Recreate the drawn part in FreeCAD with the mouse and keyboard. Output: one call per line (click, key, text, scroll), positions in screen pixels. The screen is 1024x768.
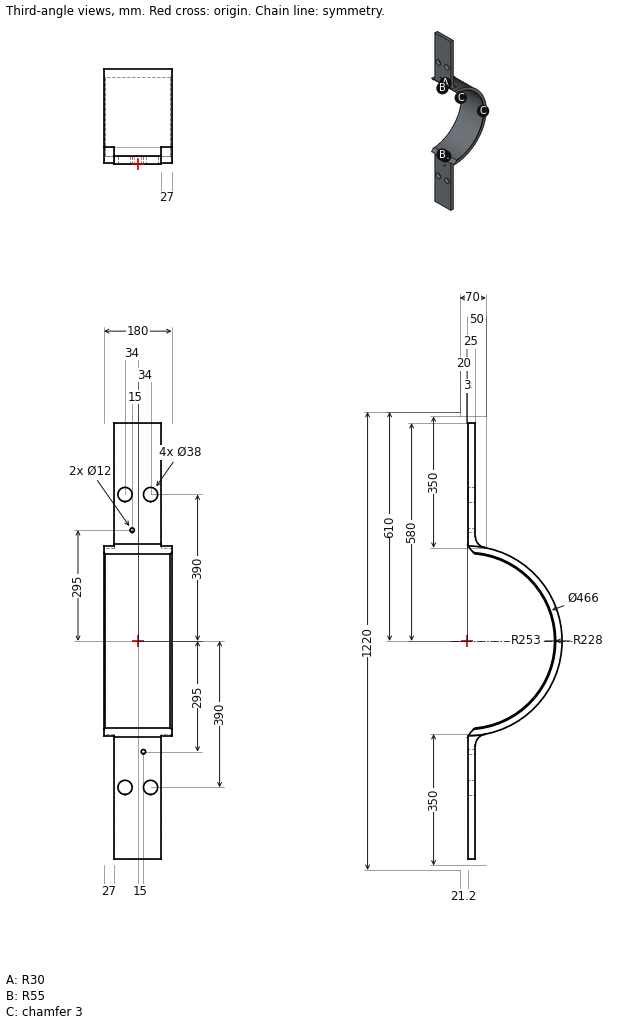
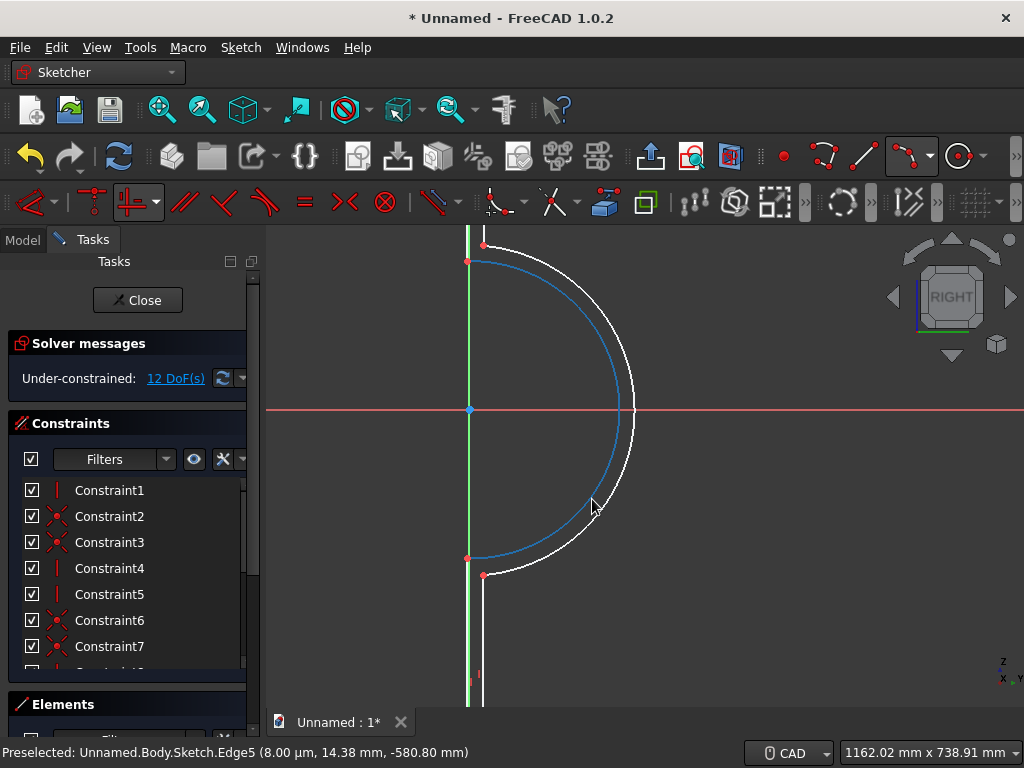
click(590, 498)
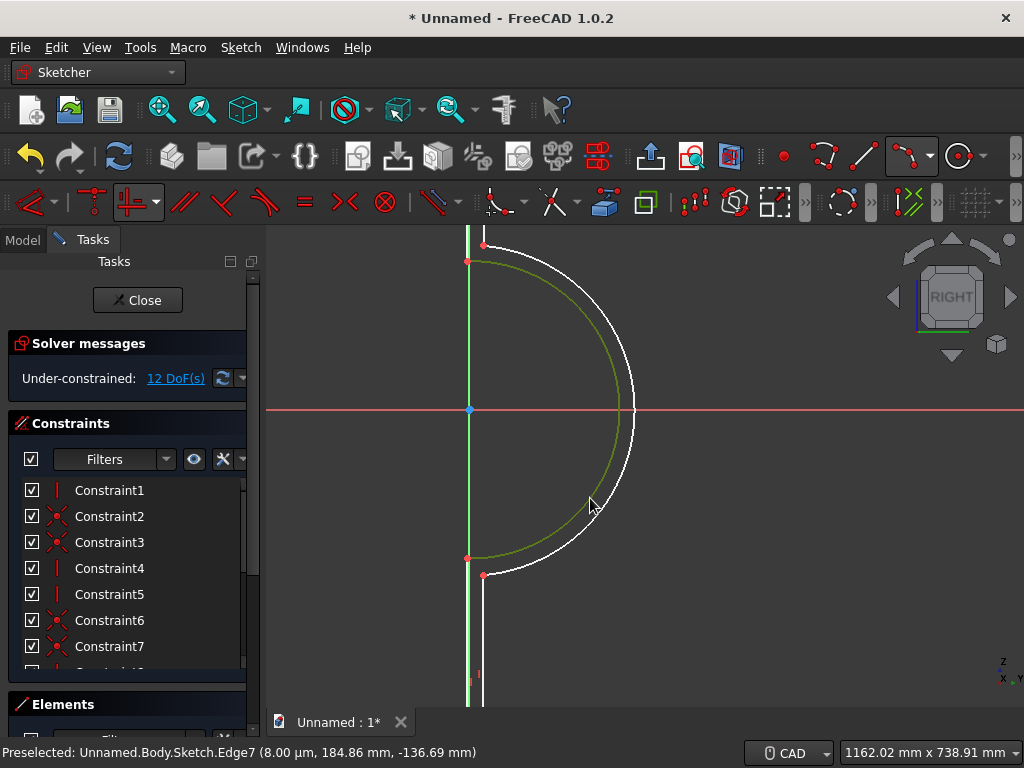
click(606, 503)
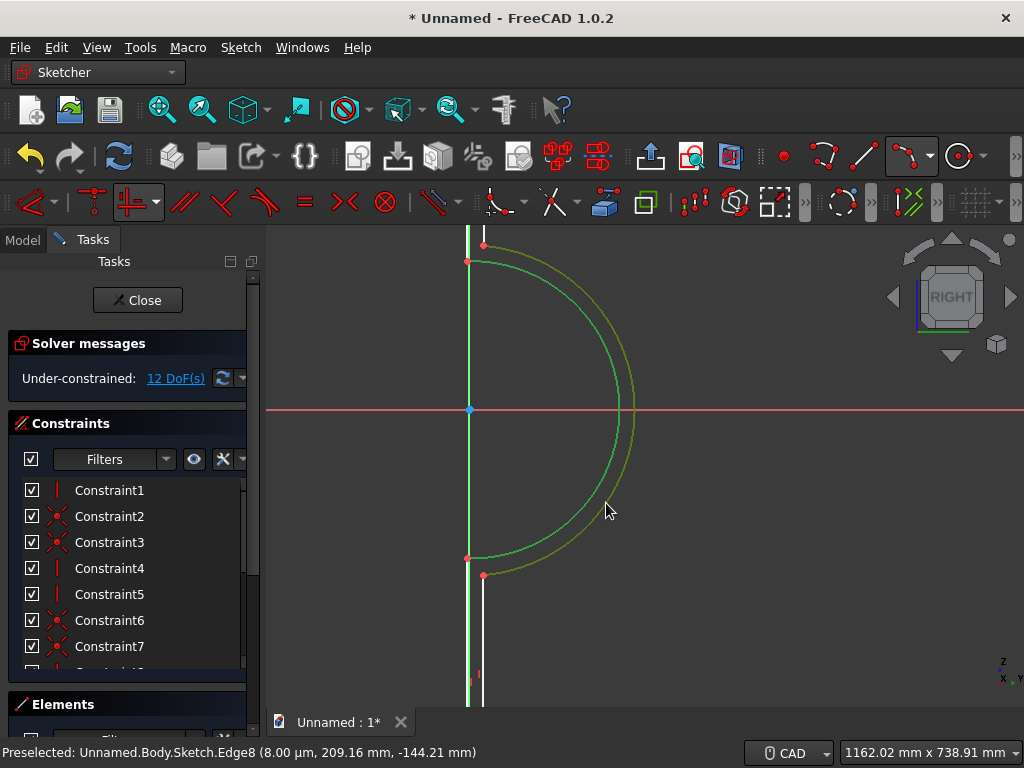
click(92, 202)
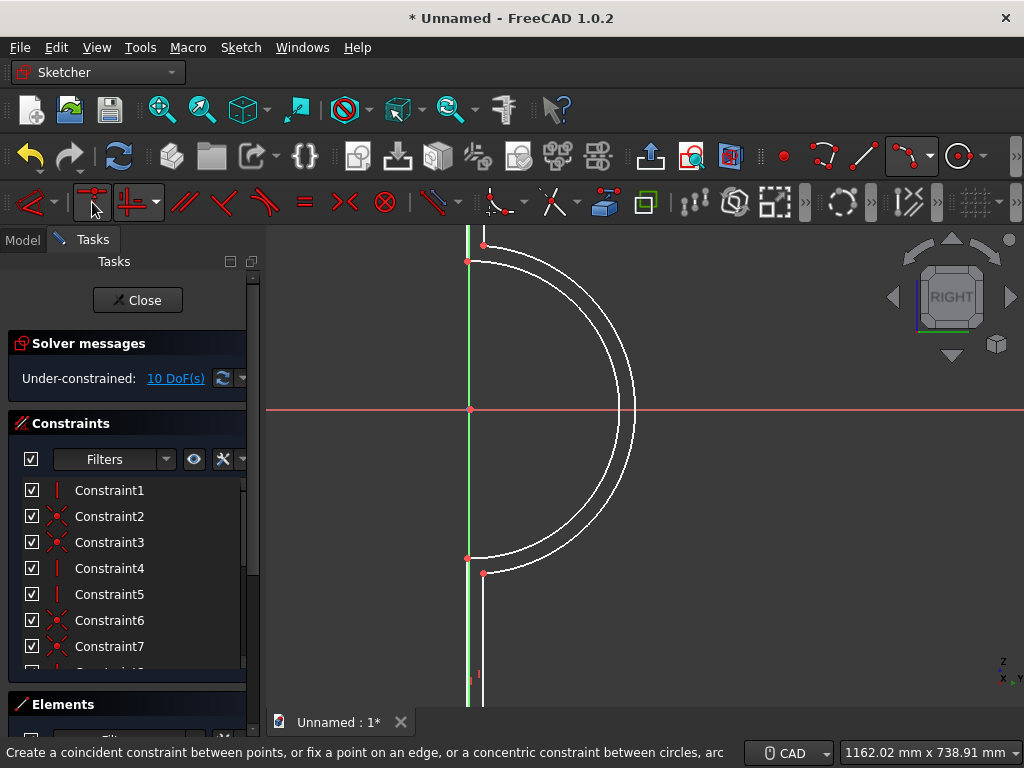
drag(459, 400, 481, 420)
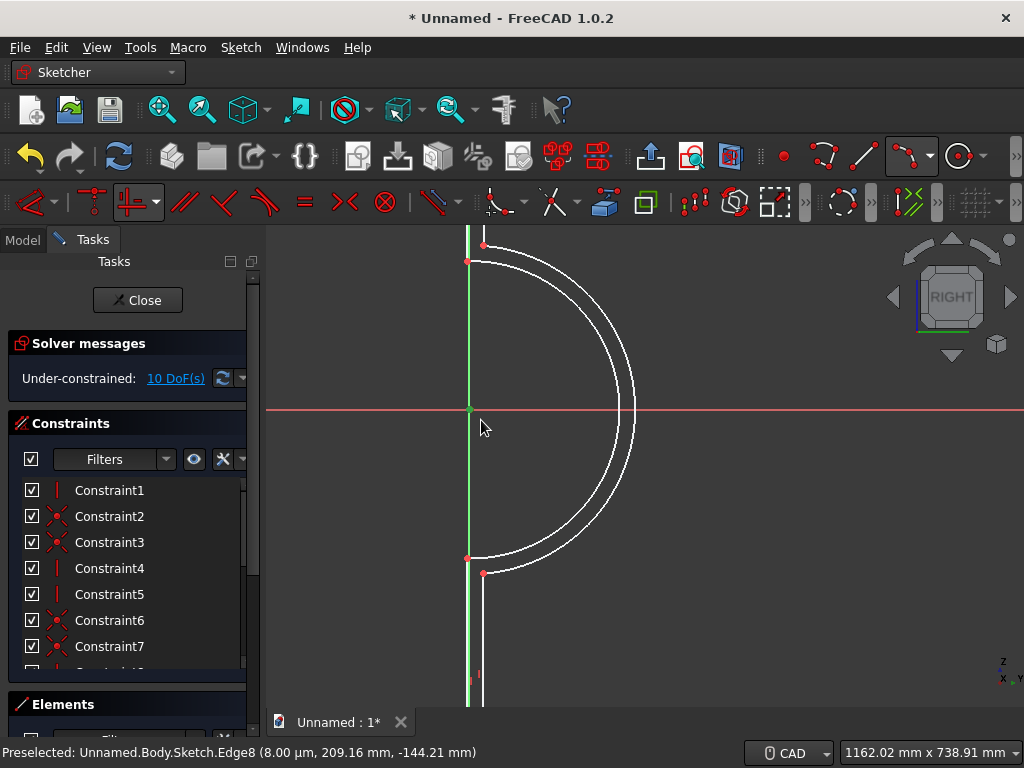
click(92, 202)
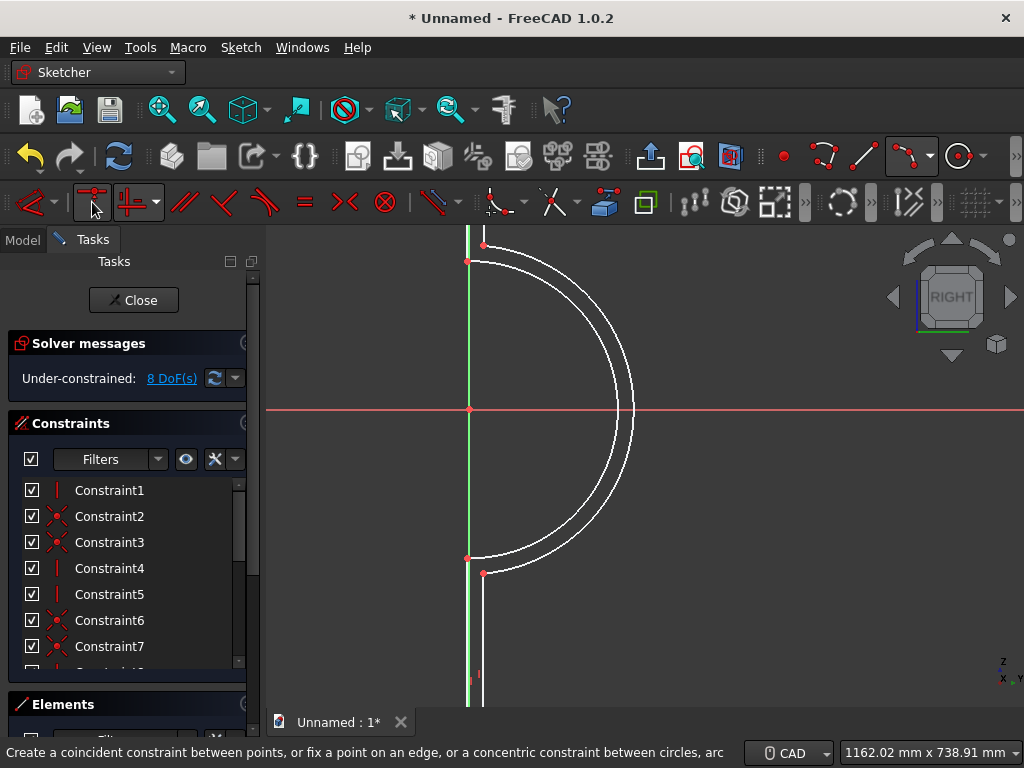
scroll(591, 499, down, 5)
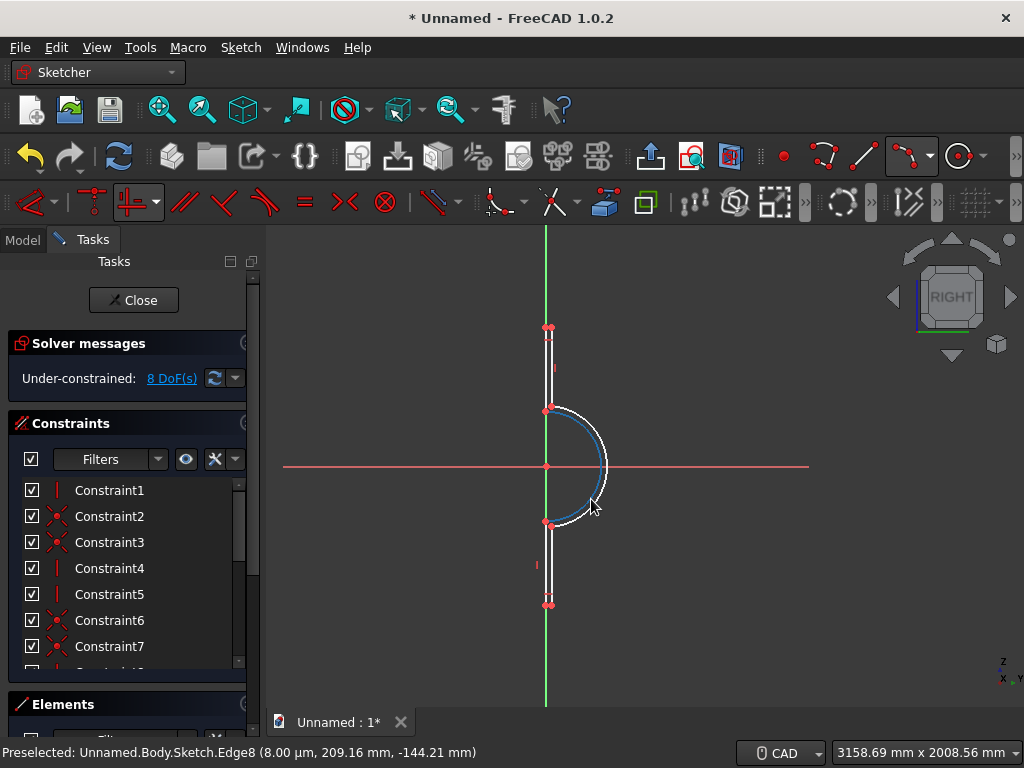
scroll(546, 328, up, 4)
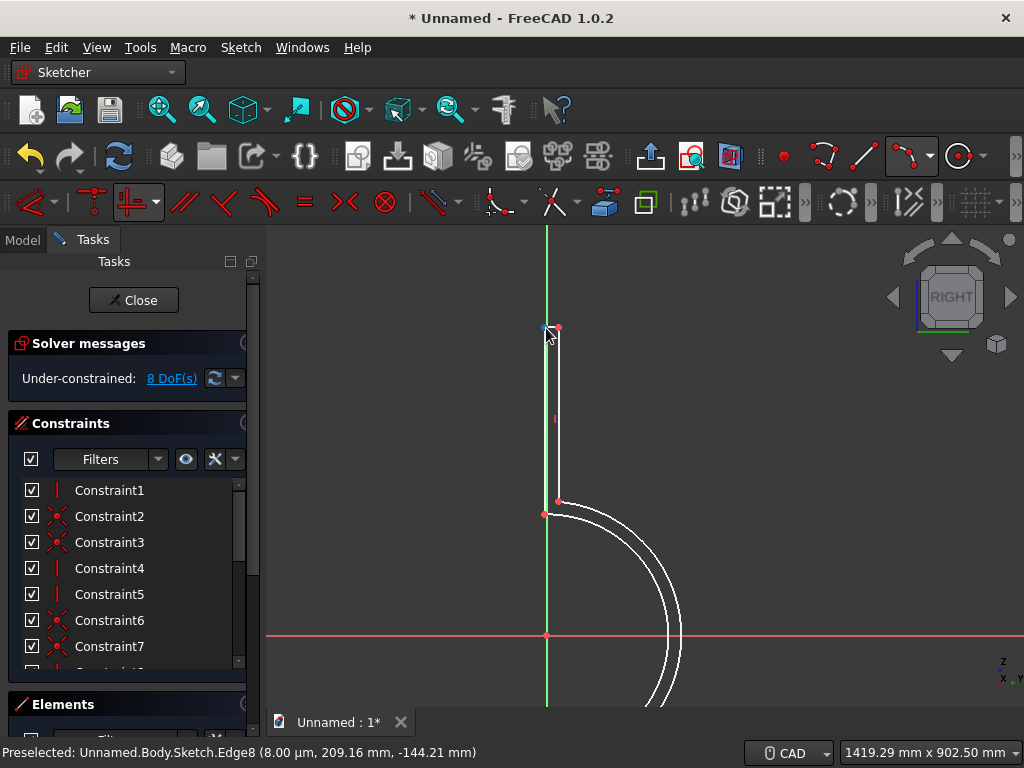
click(545, 327)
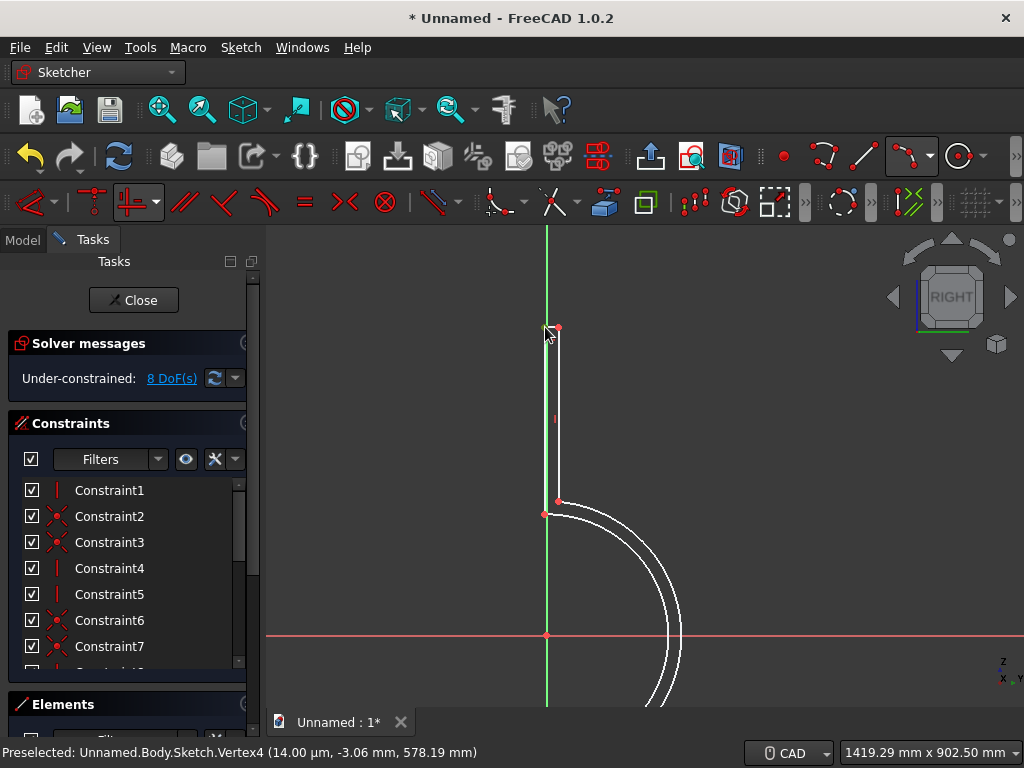
scroll(546, 327, down, 4)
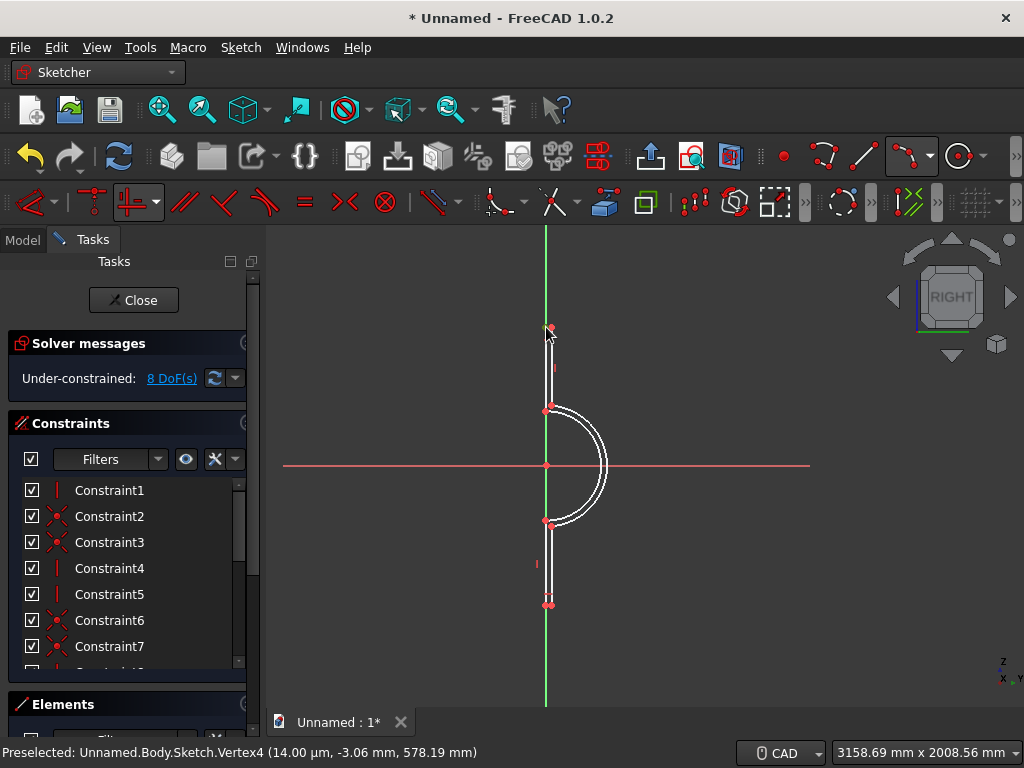
scroll(546, 605, up, 4)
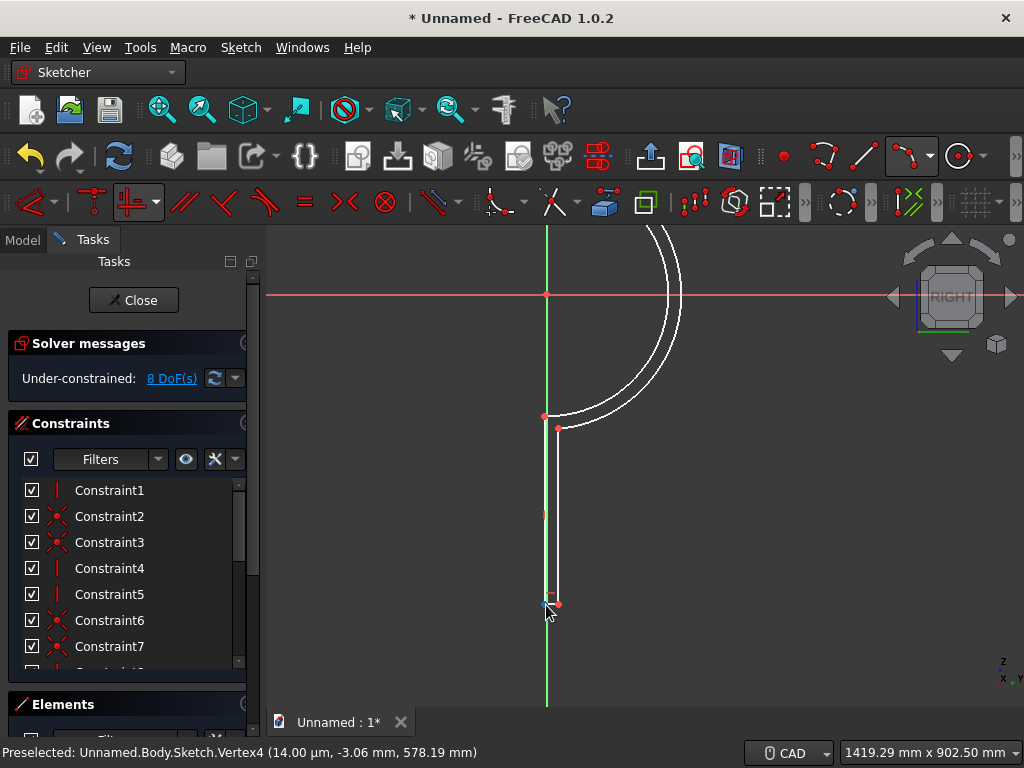
click(545, 604)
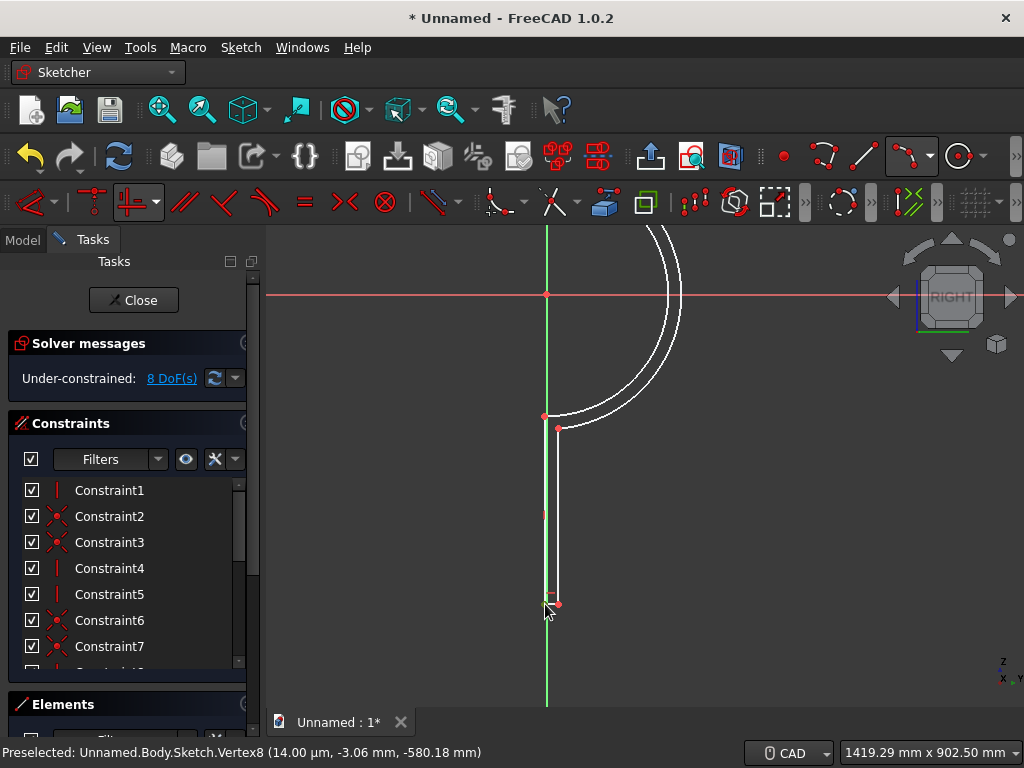
click(334, 295)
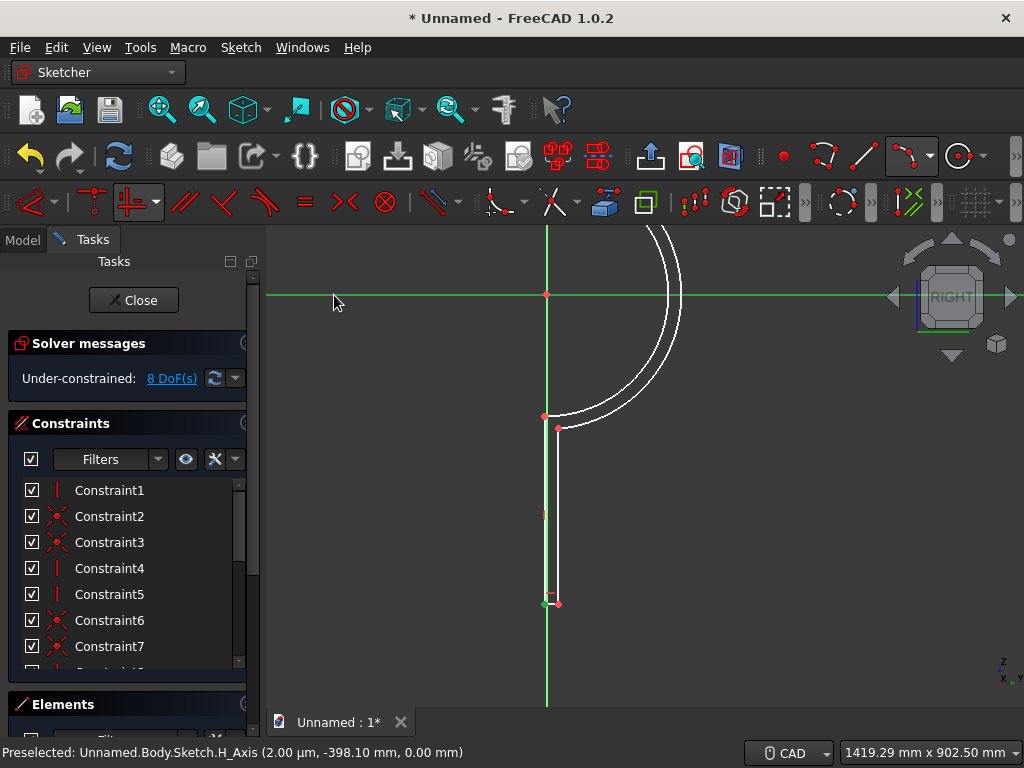
click(346, 202)